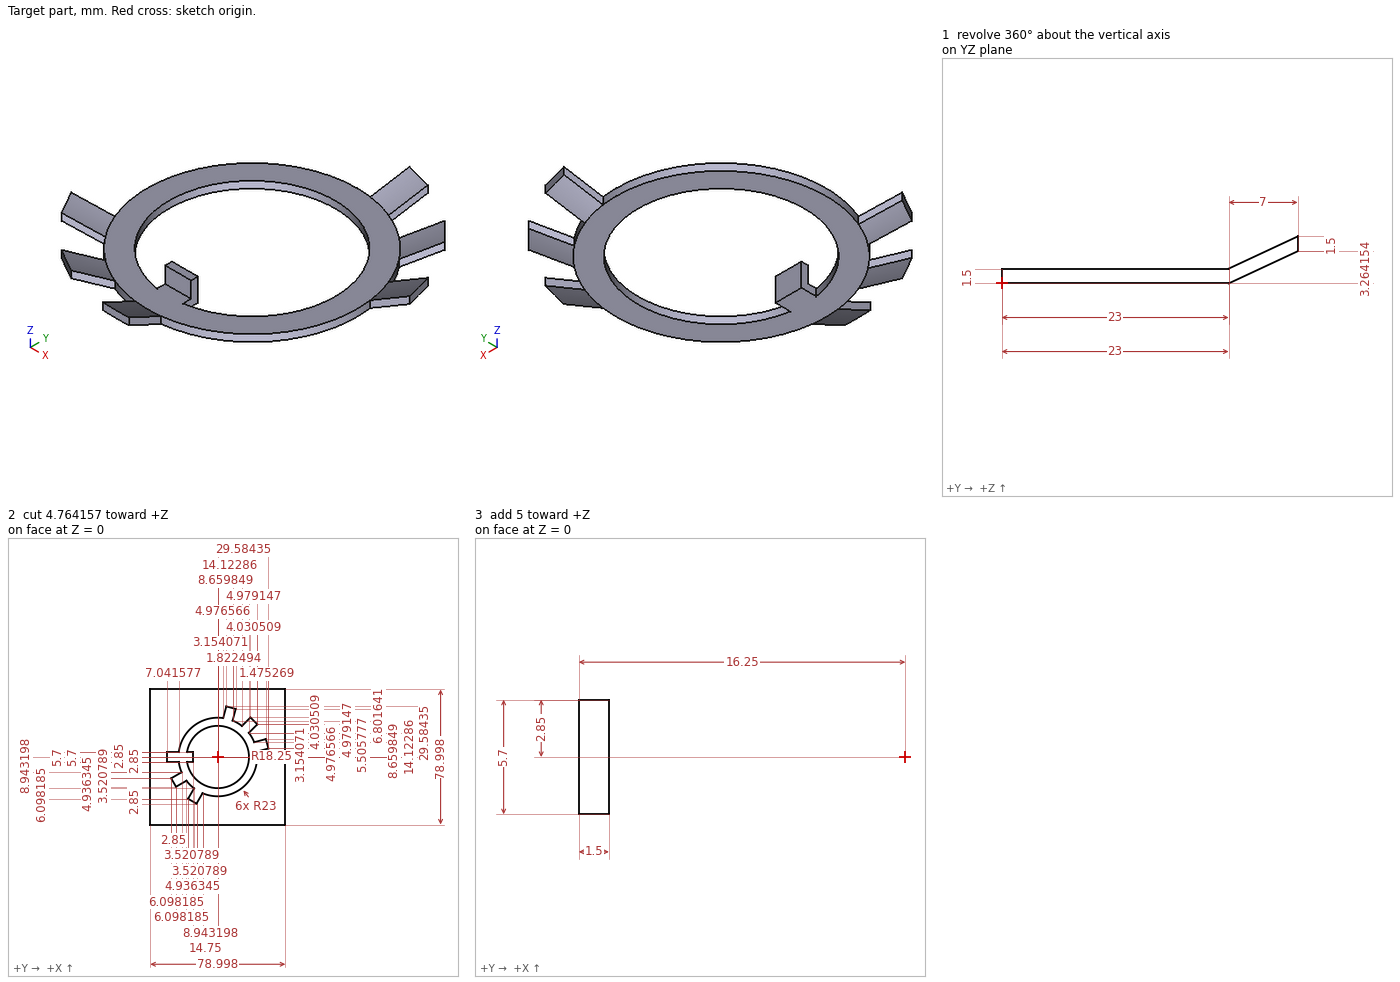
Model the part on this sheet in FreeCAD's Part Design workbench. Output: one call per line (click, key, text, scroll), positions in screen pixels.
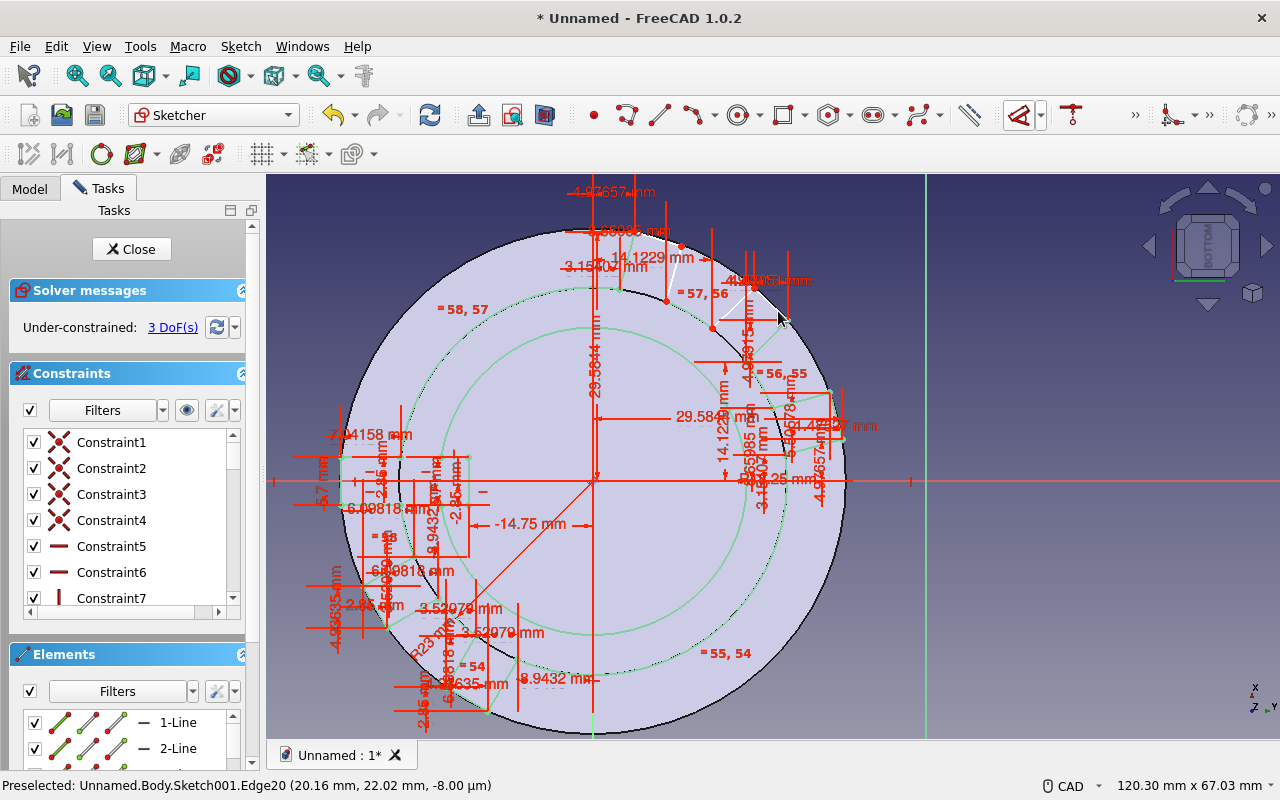
click(778, 311)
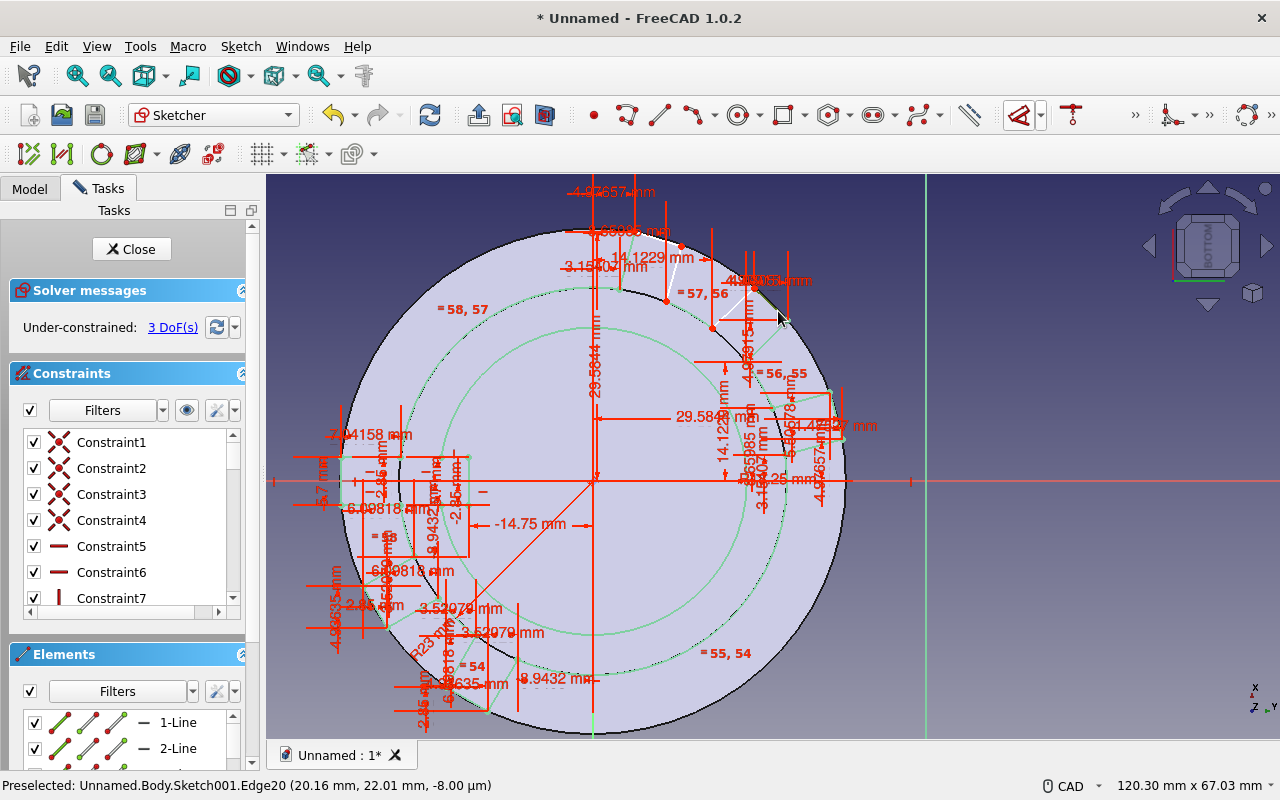
key(i)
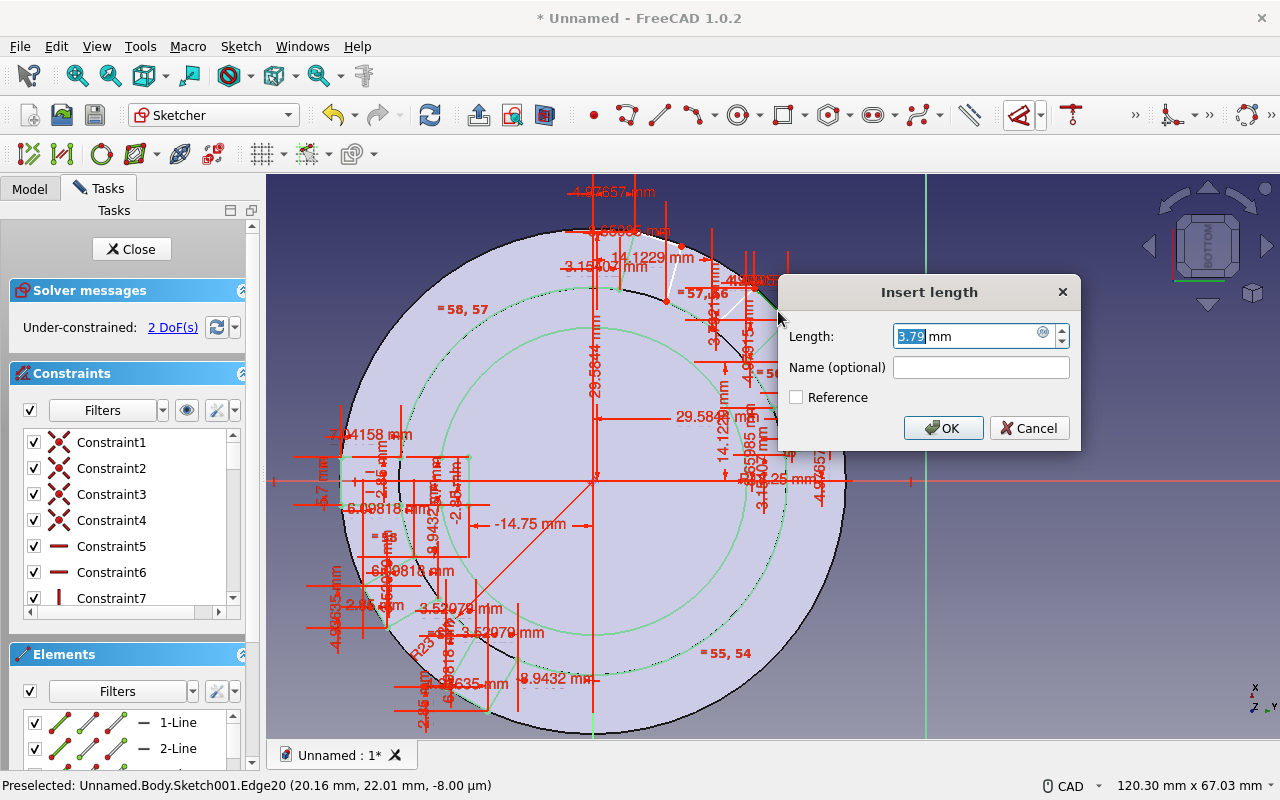
text(4.030509)
key(Return)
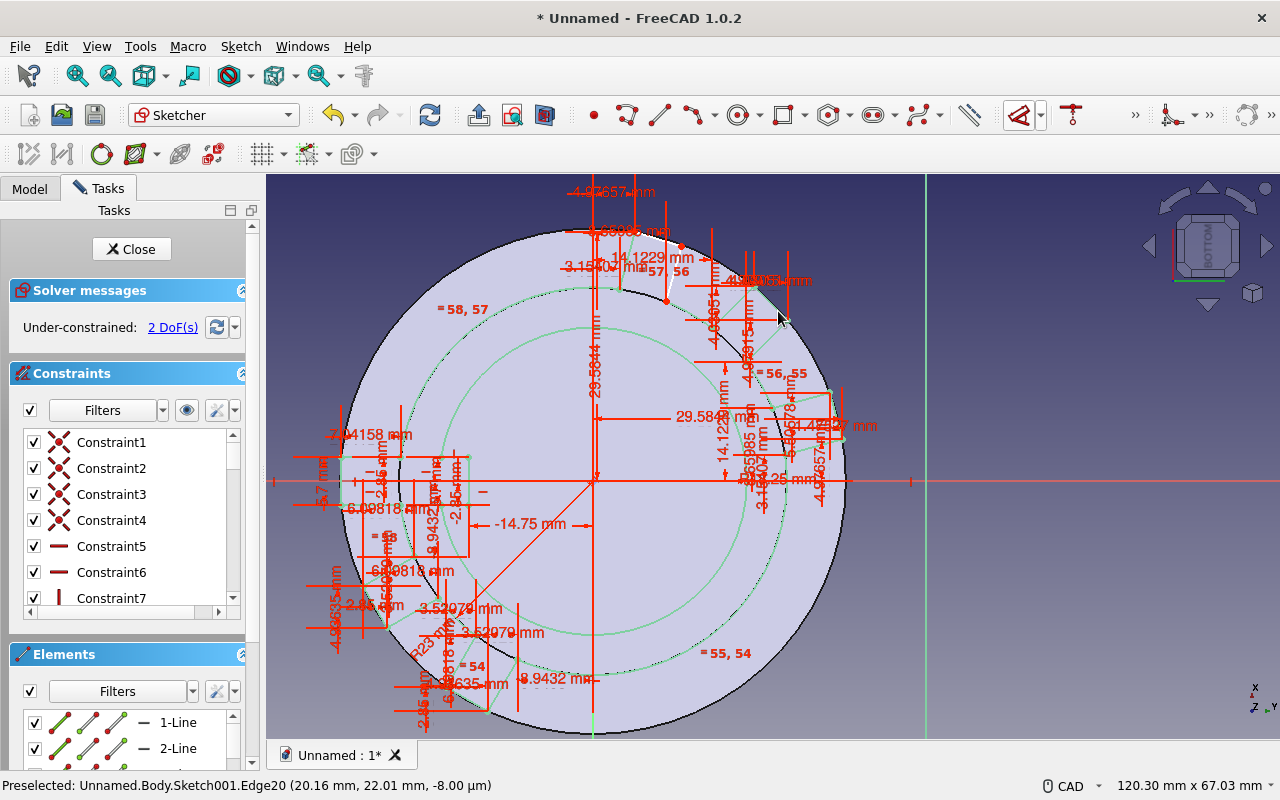
scroll(671, 285, up, 5)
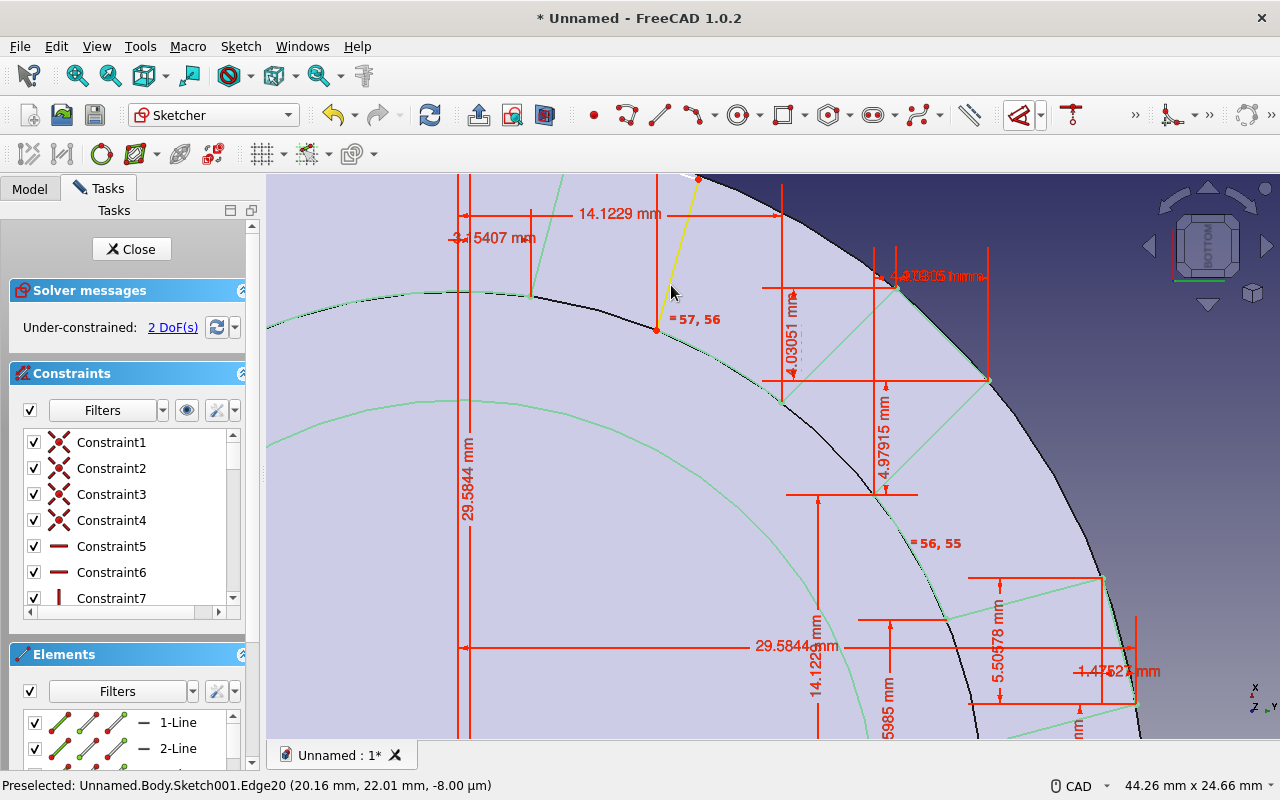
click(669, 285)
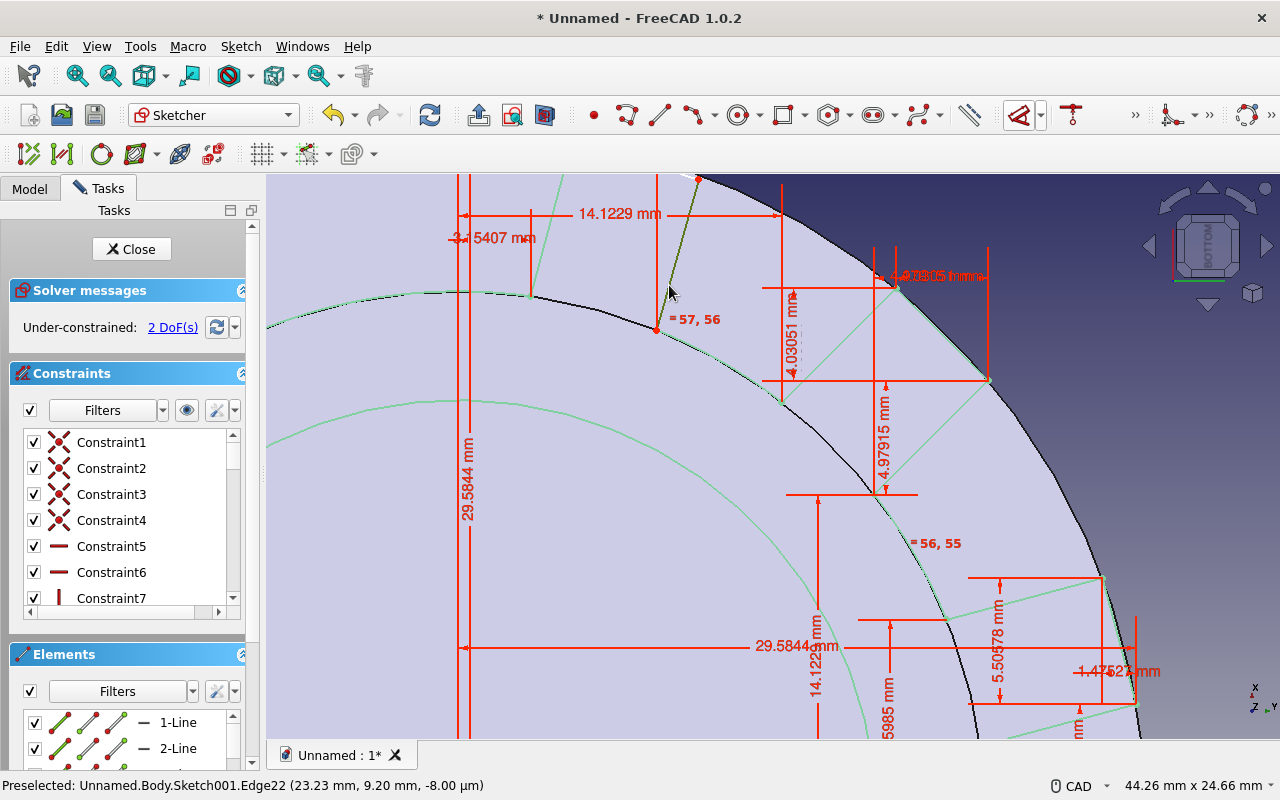
click(1040, 116)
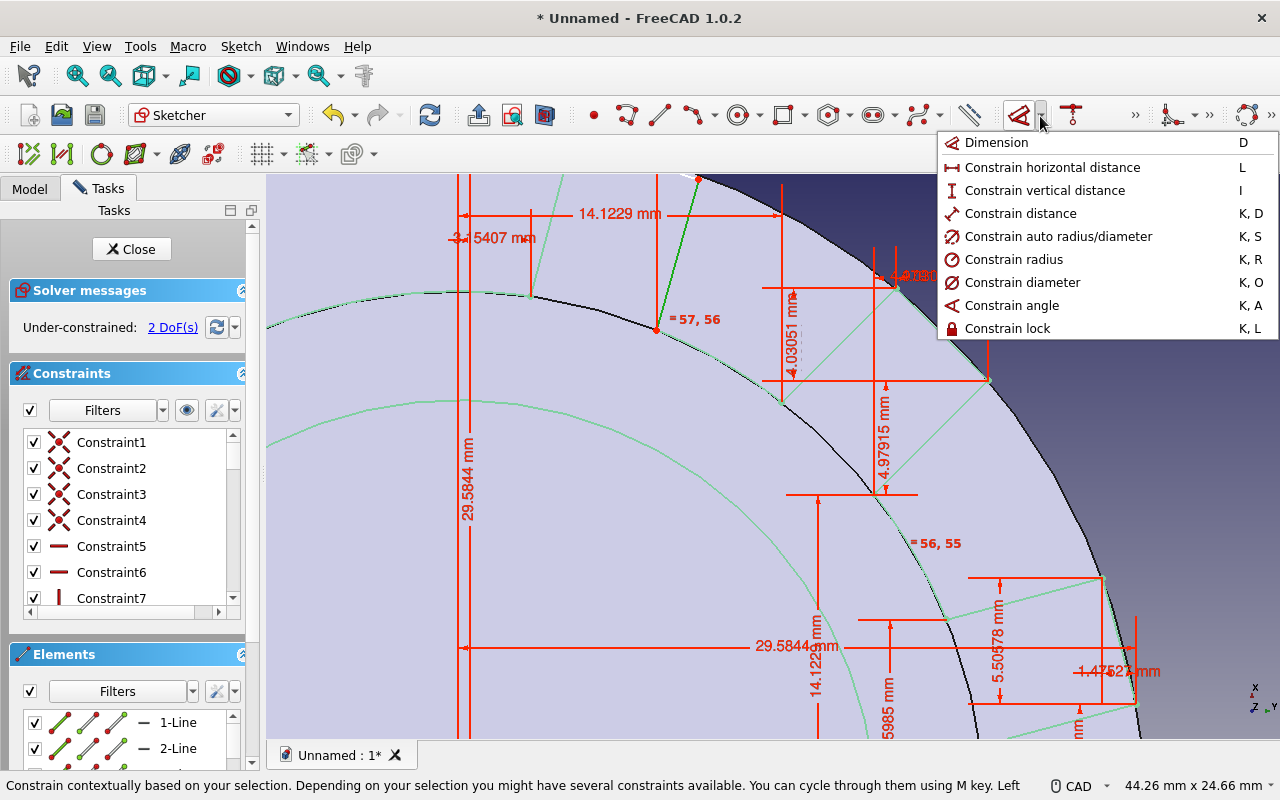
click(1108, 168)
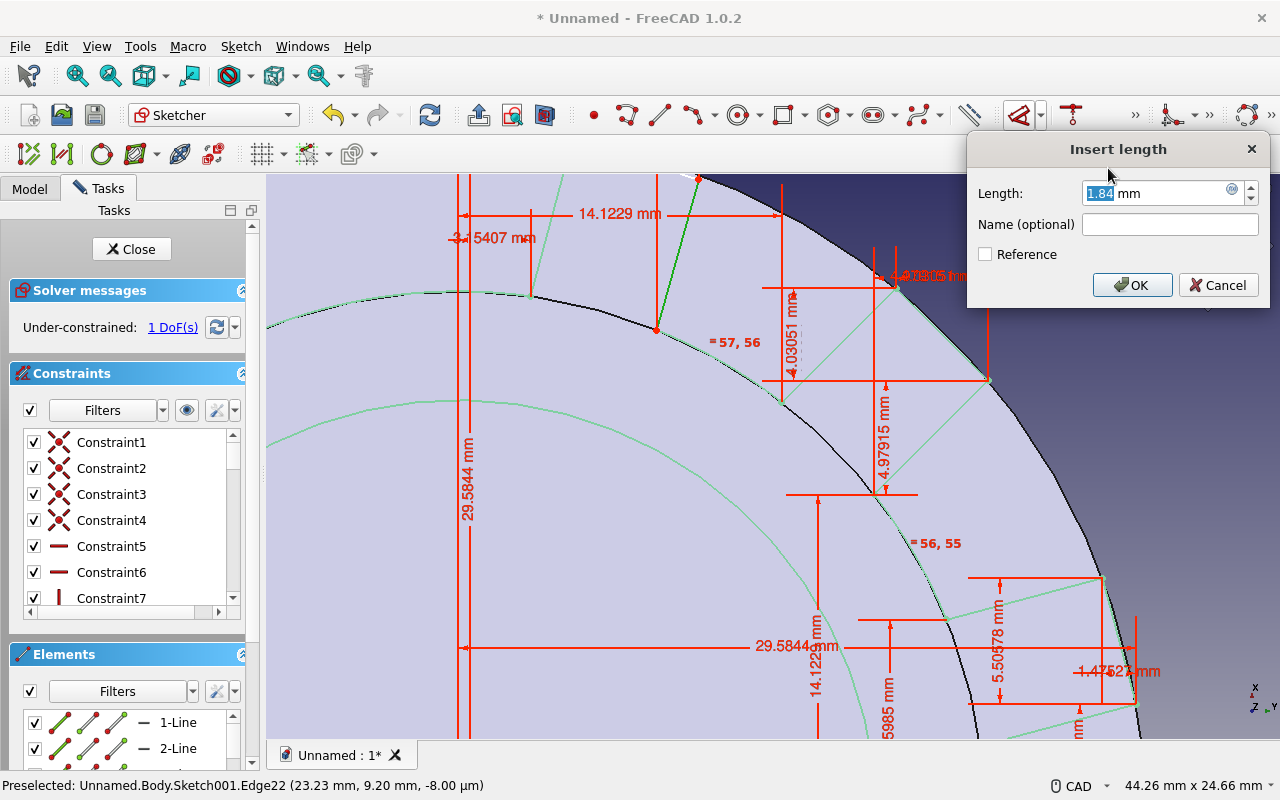
text(1.822494)
key(Return)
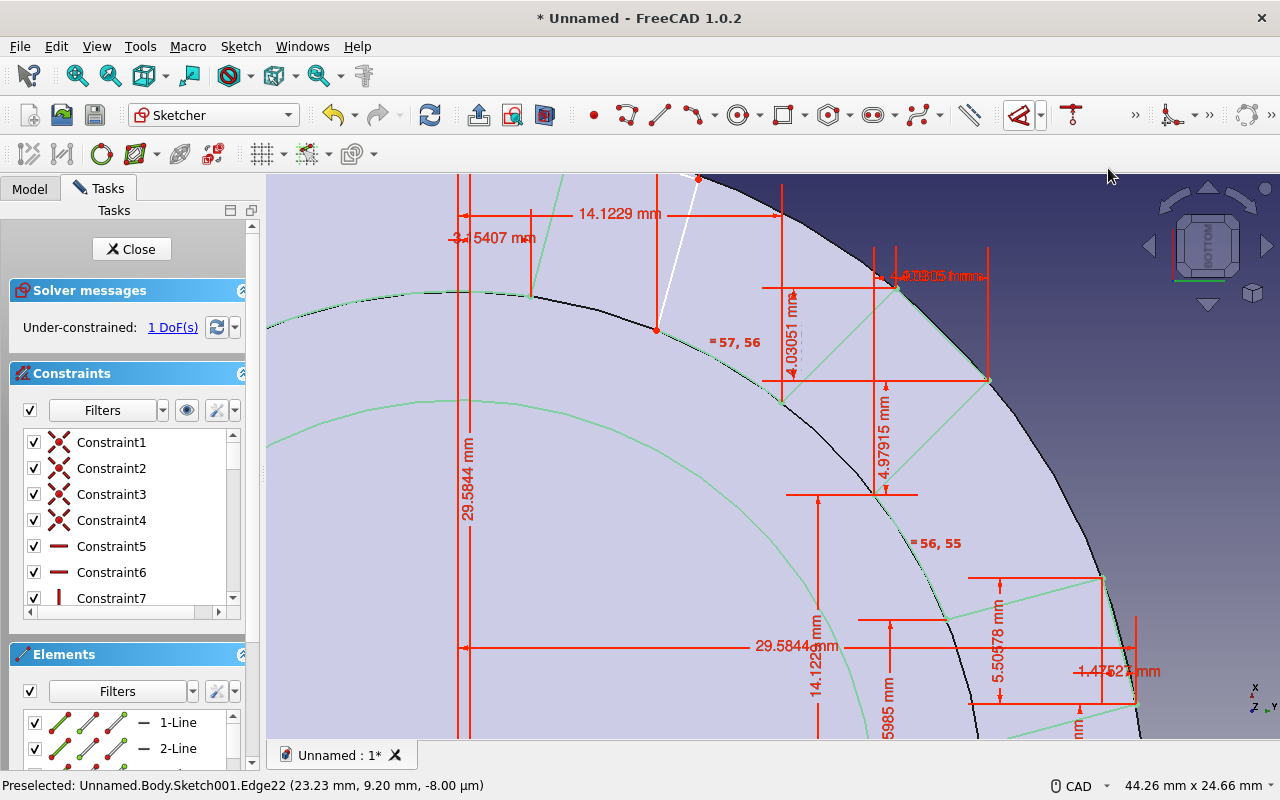
scroll(767, 365, down, 8)